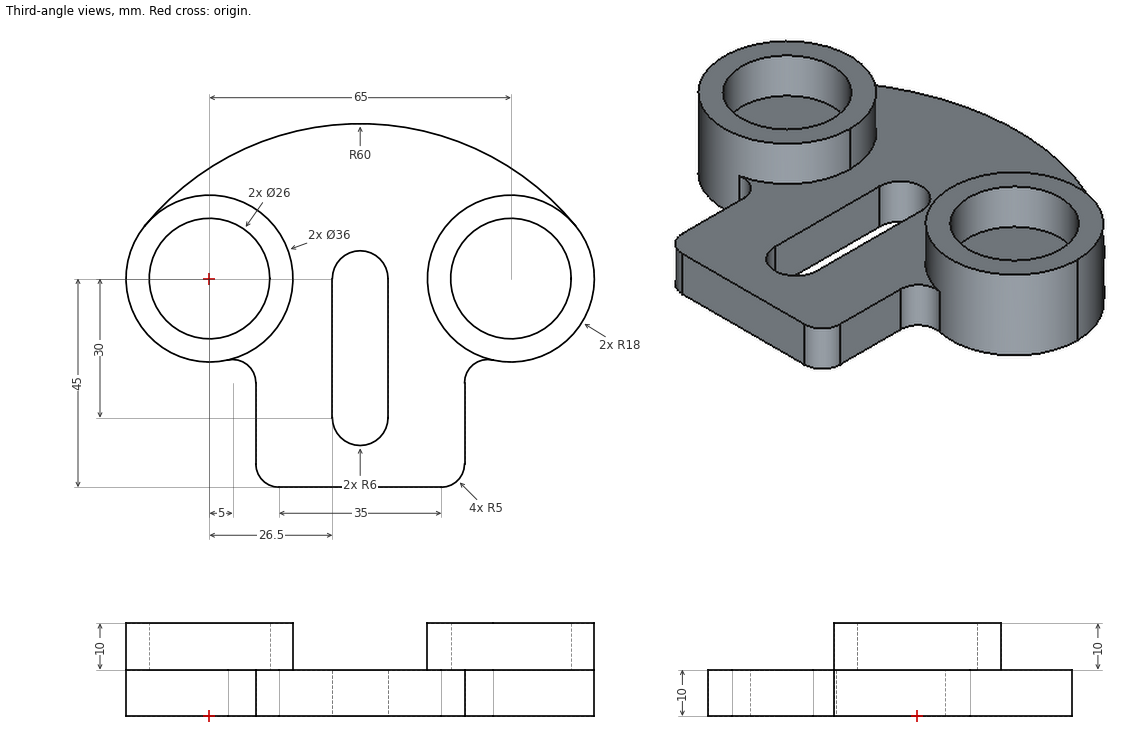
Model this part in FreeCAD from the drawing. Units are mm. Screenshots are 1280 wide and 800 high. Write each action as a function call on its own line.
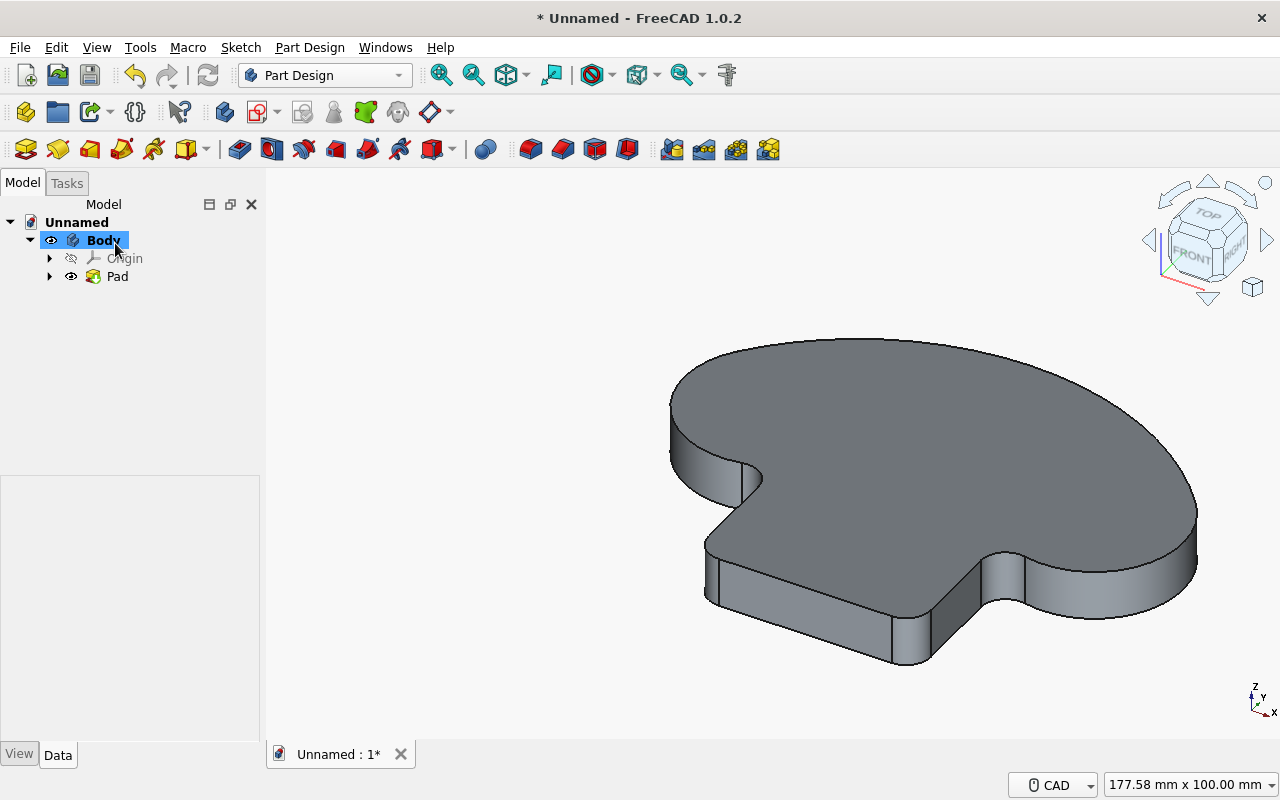
click(949, 444)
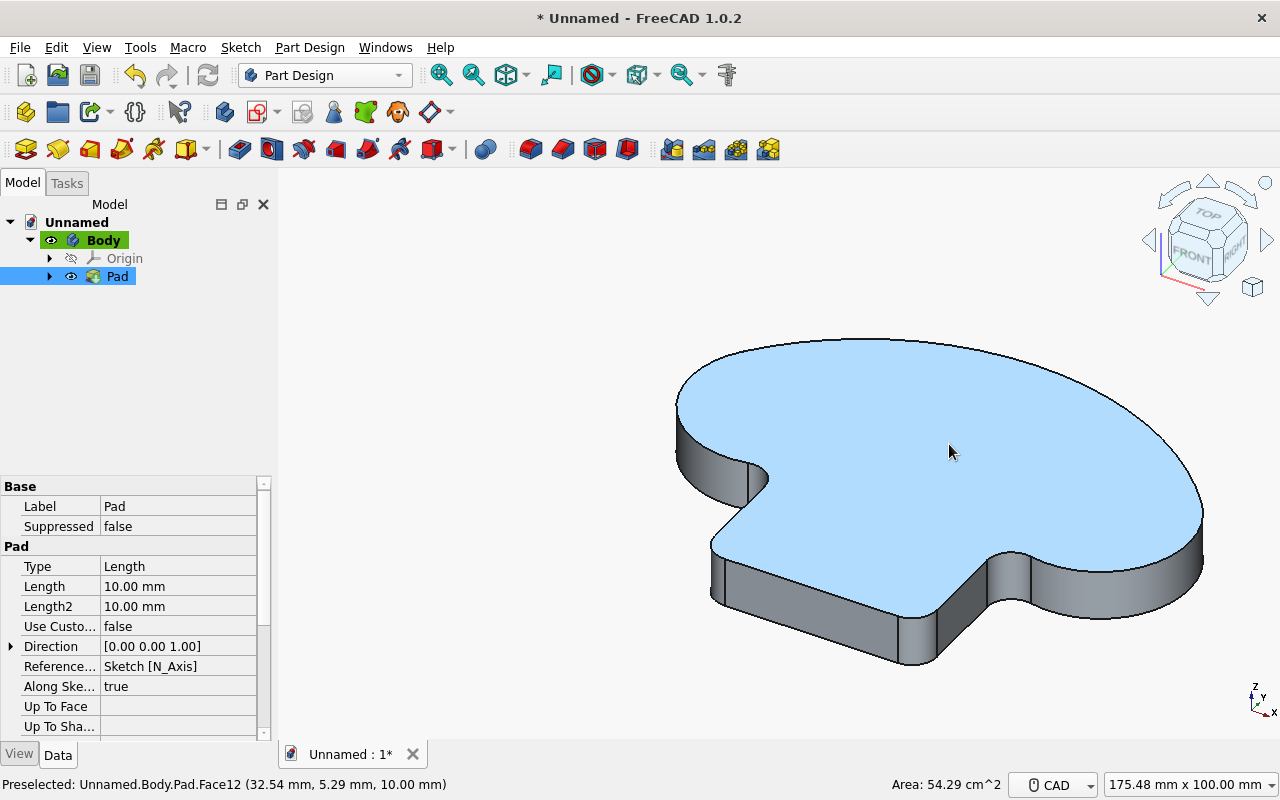
click(258, 112)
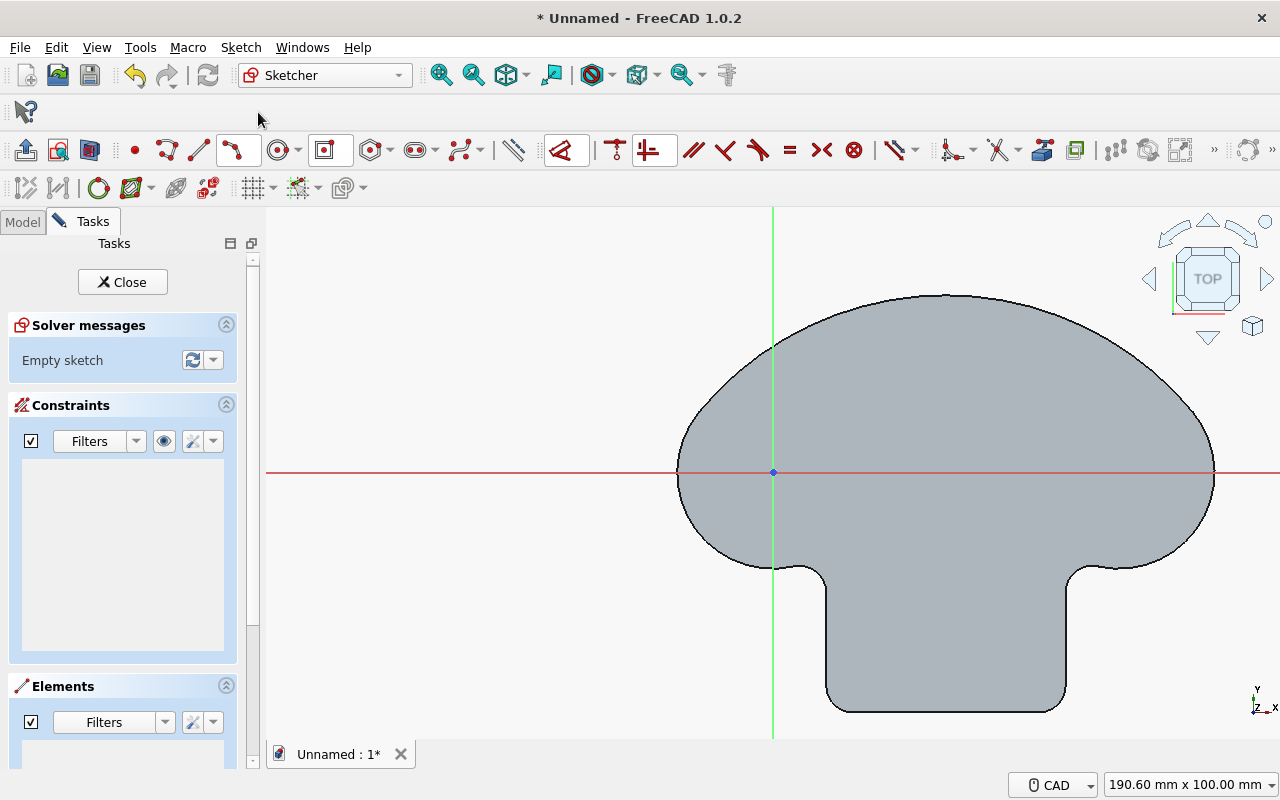
scroll(294, 473, down, 1)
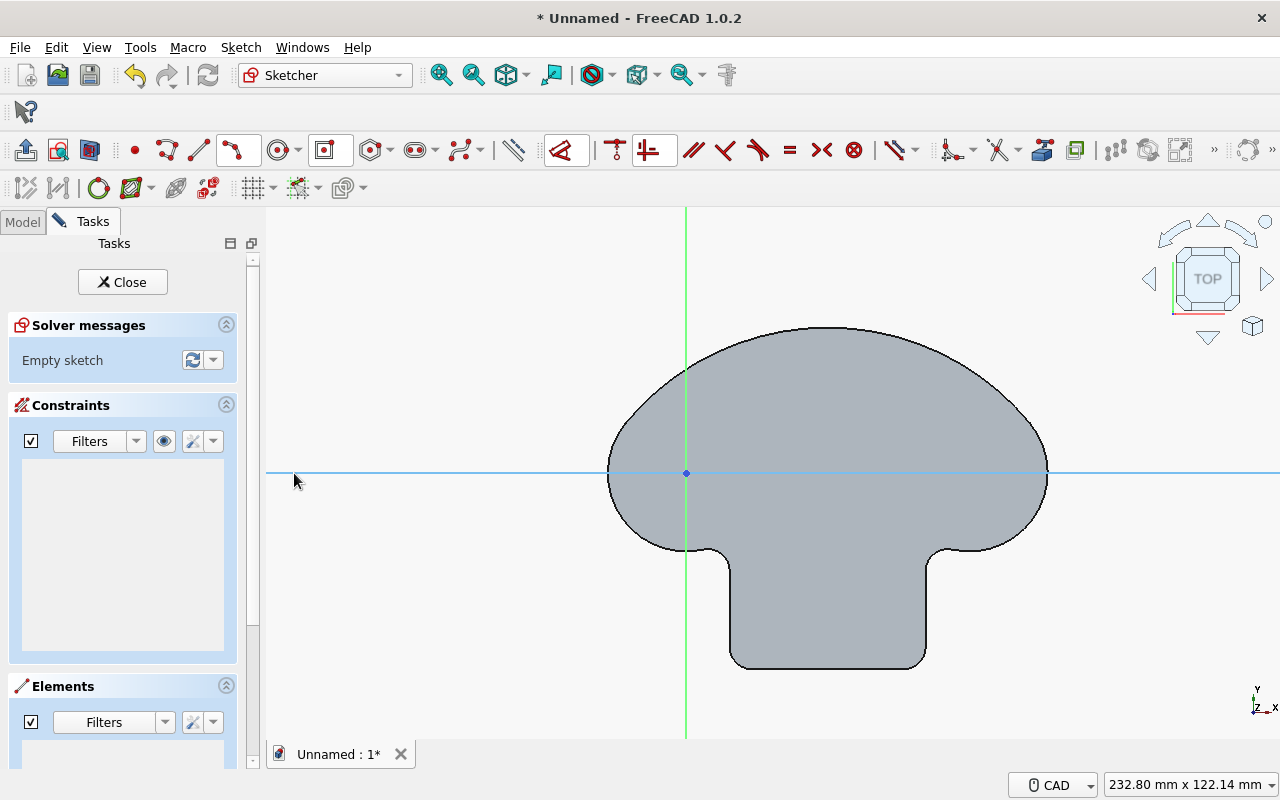
click(278, 150)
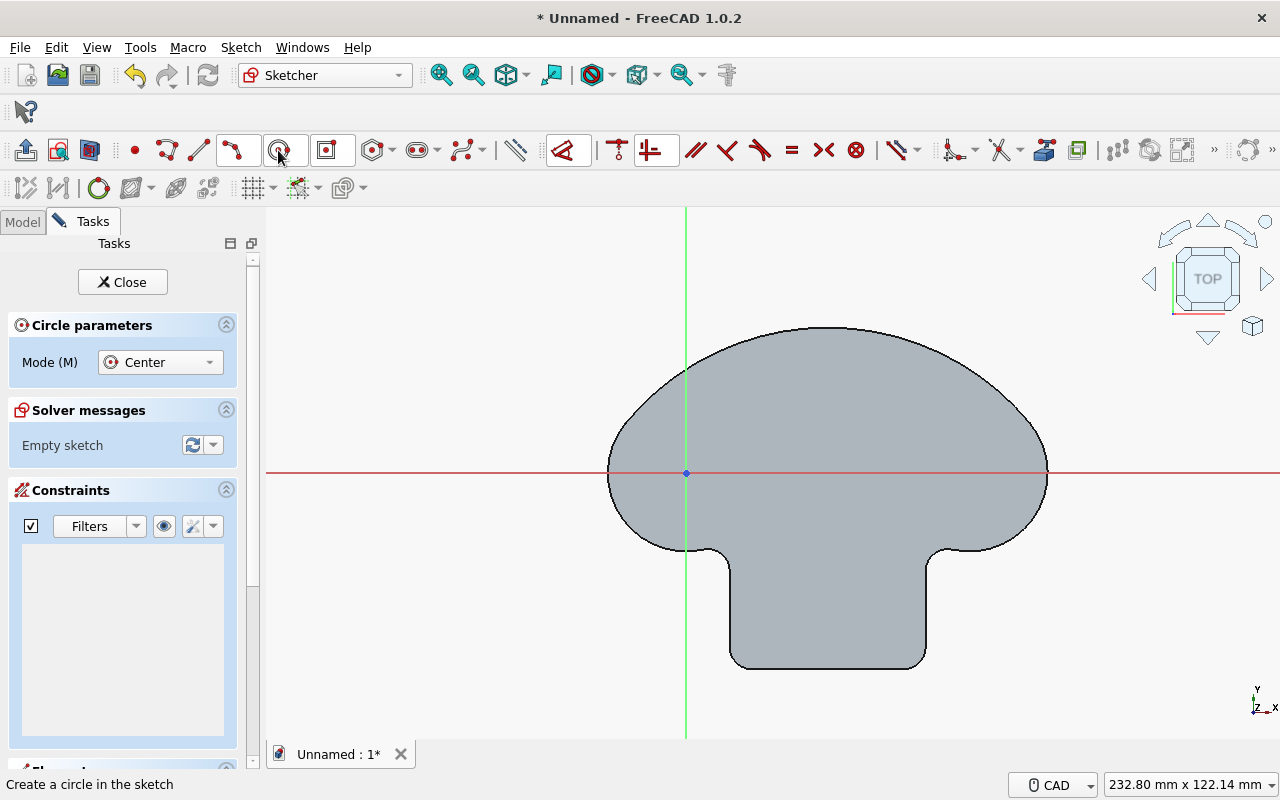
click(686, 473)
move(742, 418)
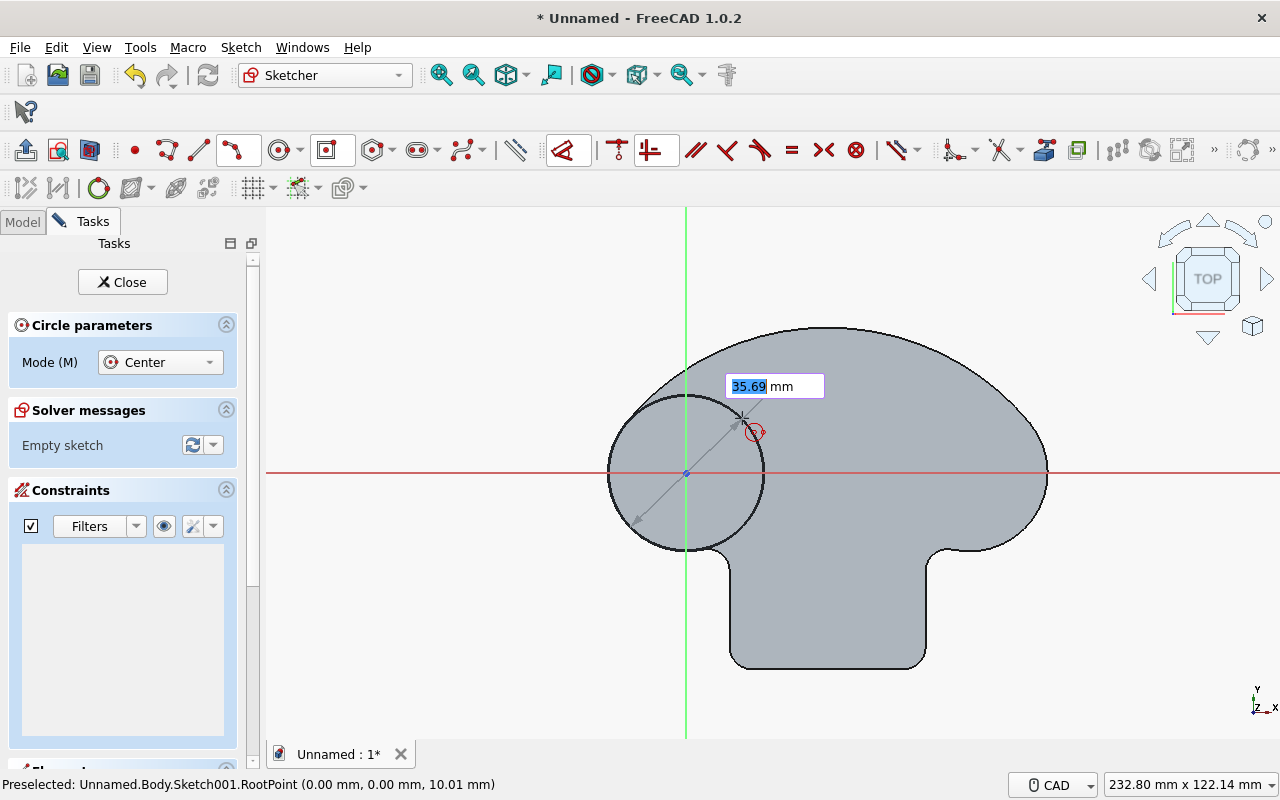
text(36)
key(Return)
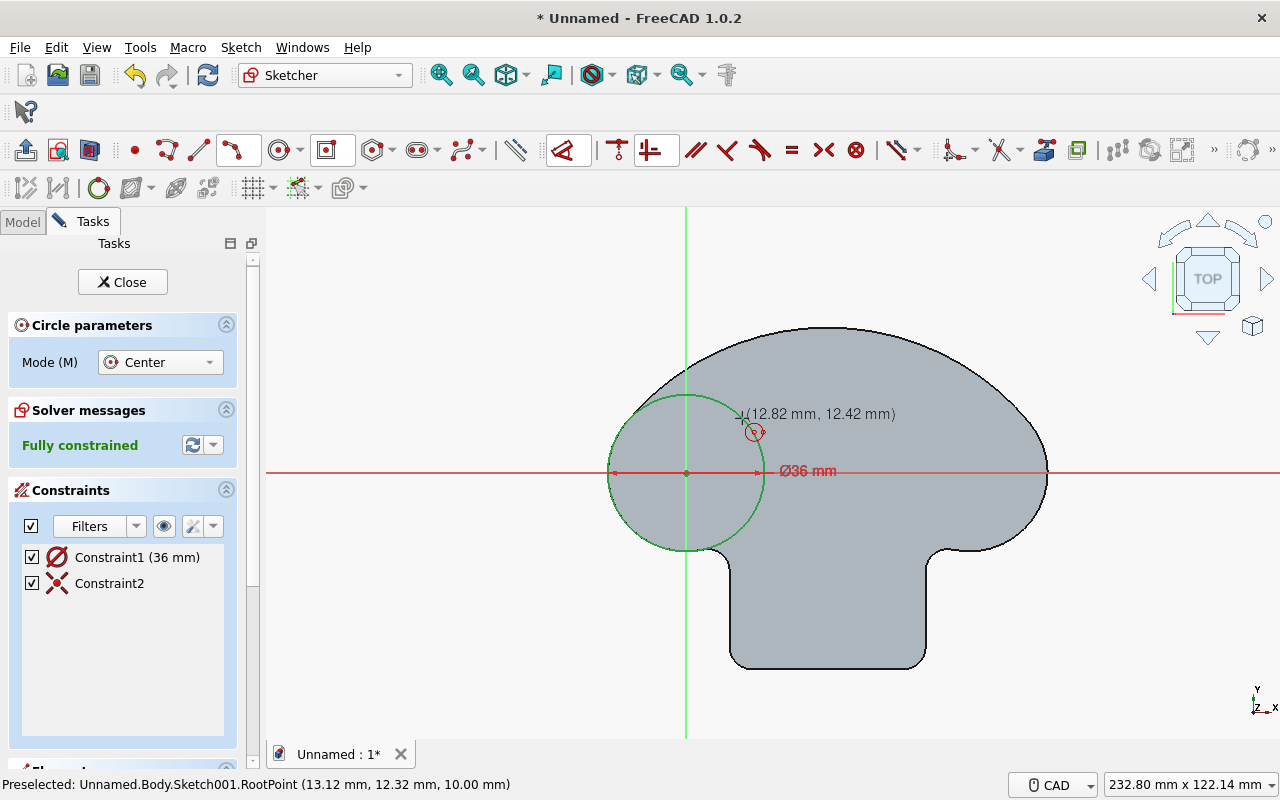
click(969, 473)
move(1025, 418)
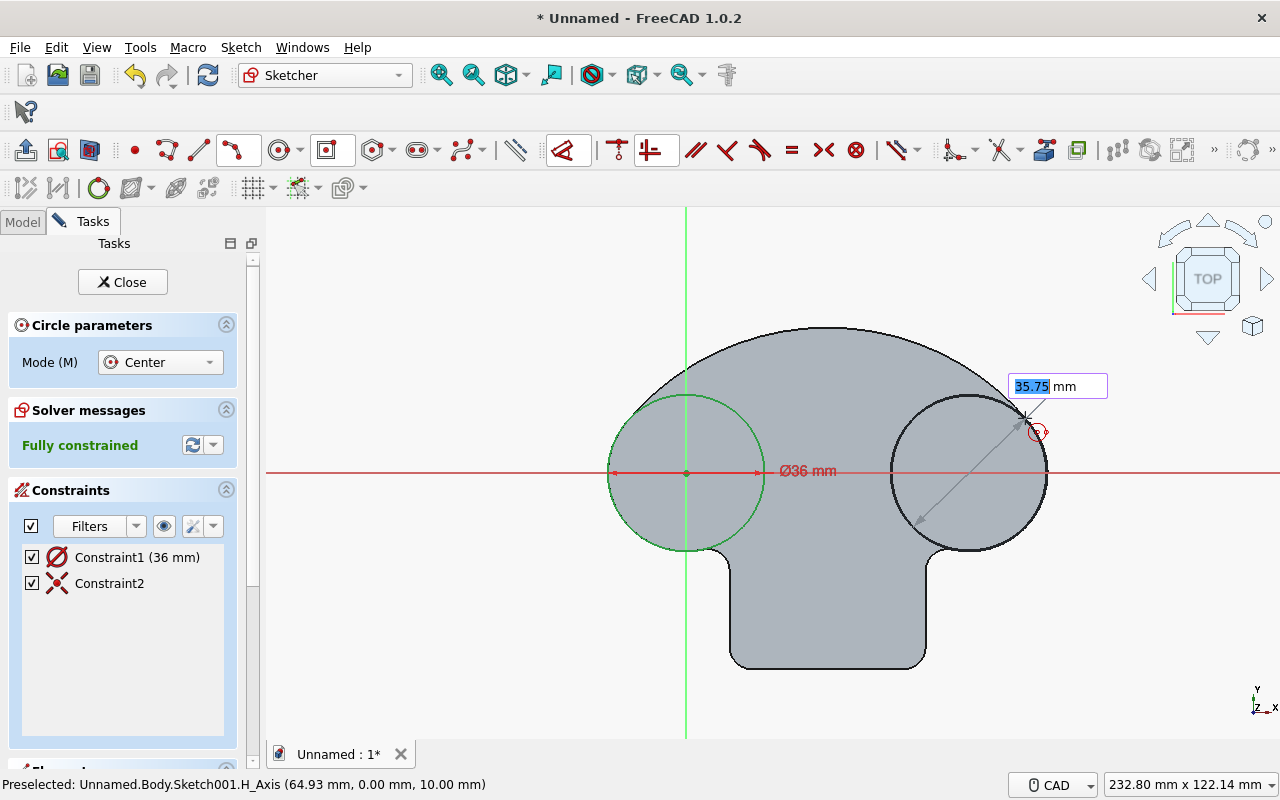
text(36)
key(Return)
key(Escape)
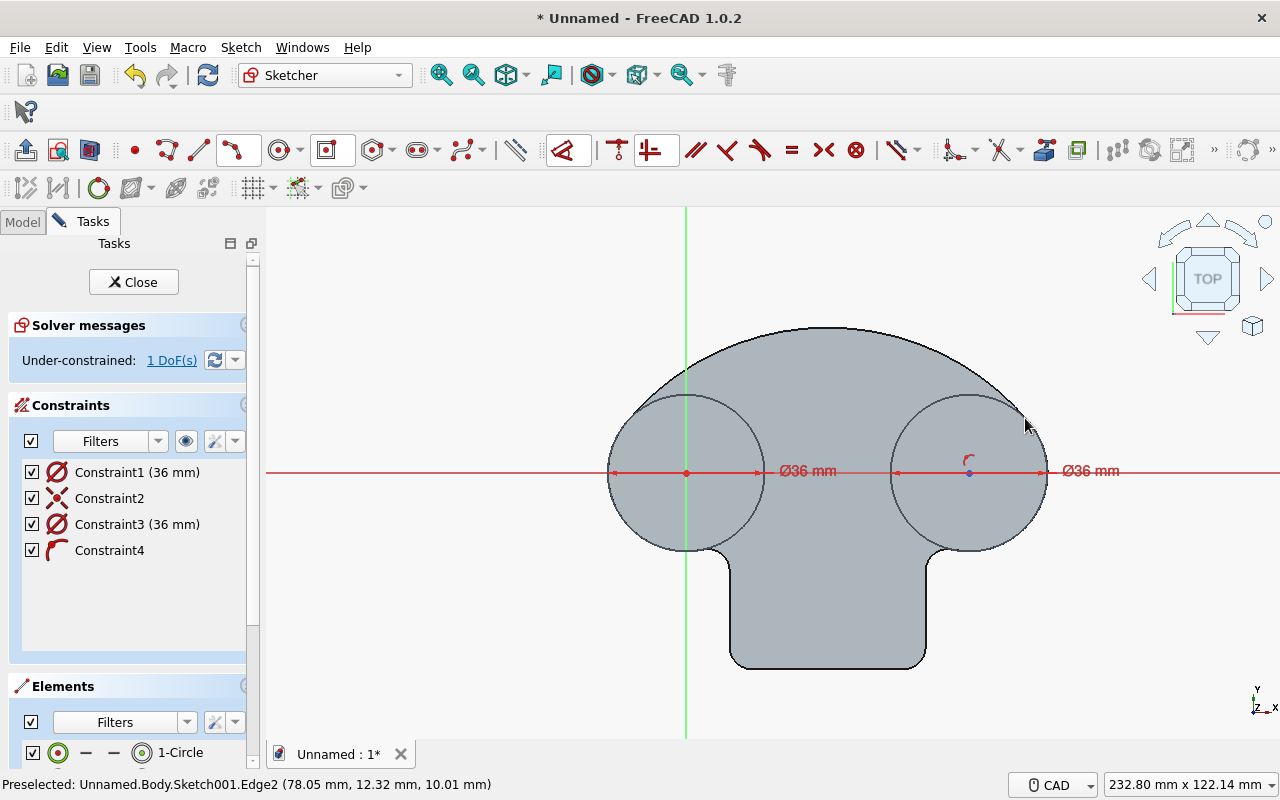
click(969, 473)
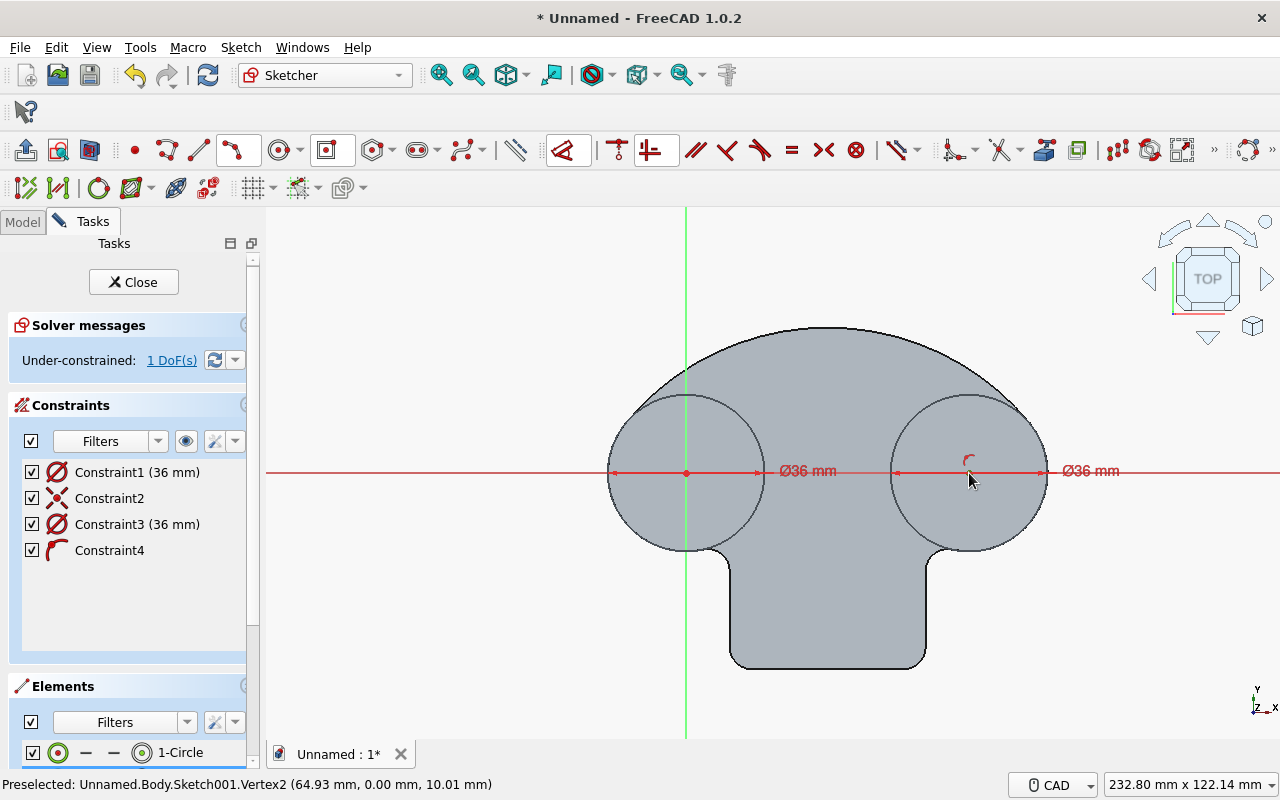
click(586, 150)